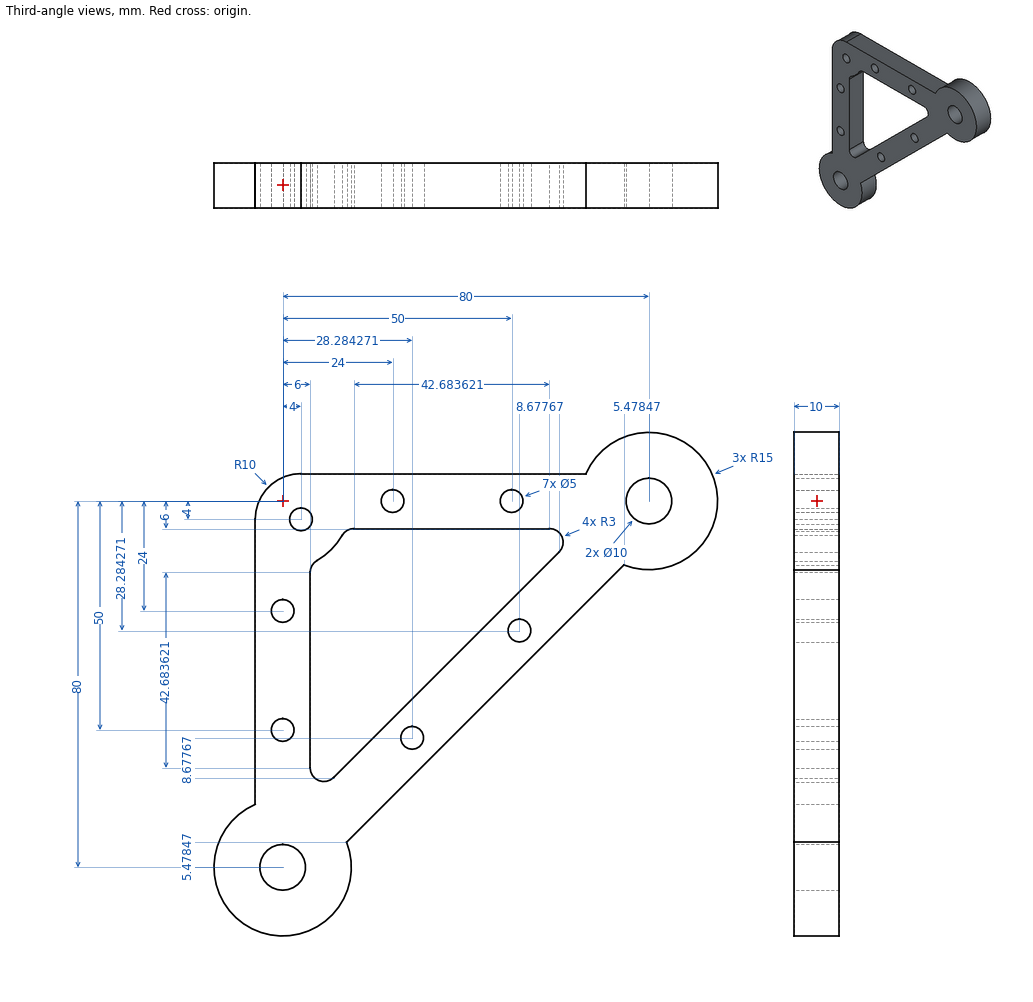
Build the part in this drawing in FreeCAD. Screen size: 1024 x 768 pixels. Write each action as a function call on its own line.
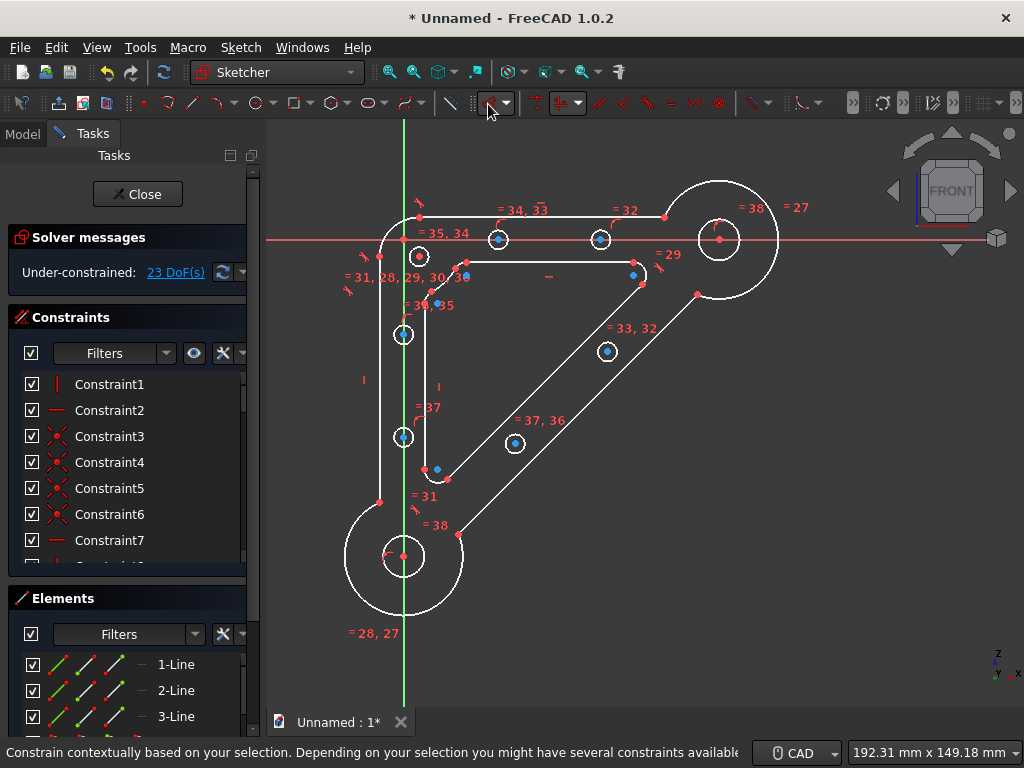
click(401, 222)
click(386, 194)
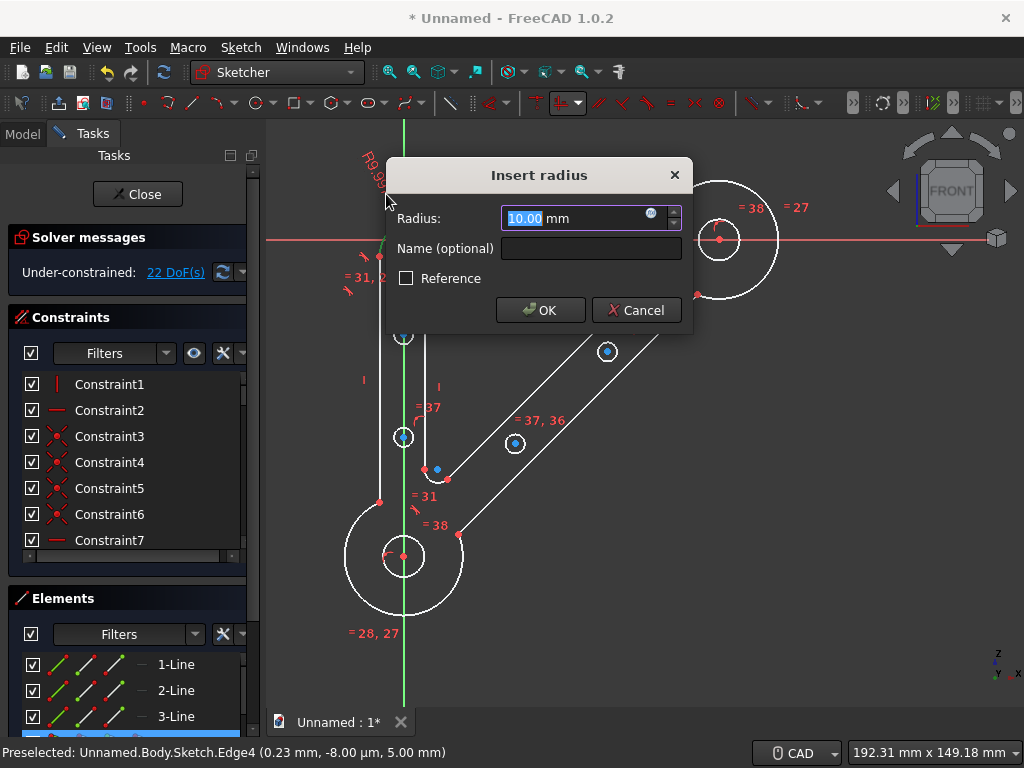
text(10)
key(Return)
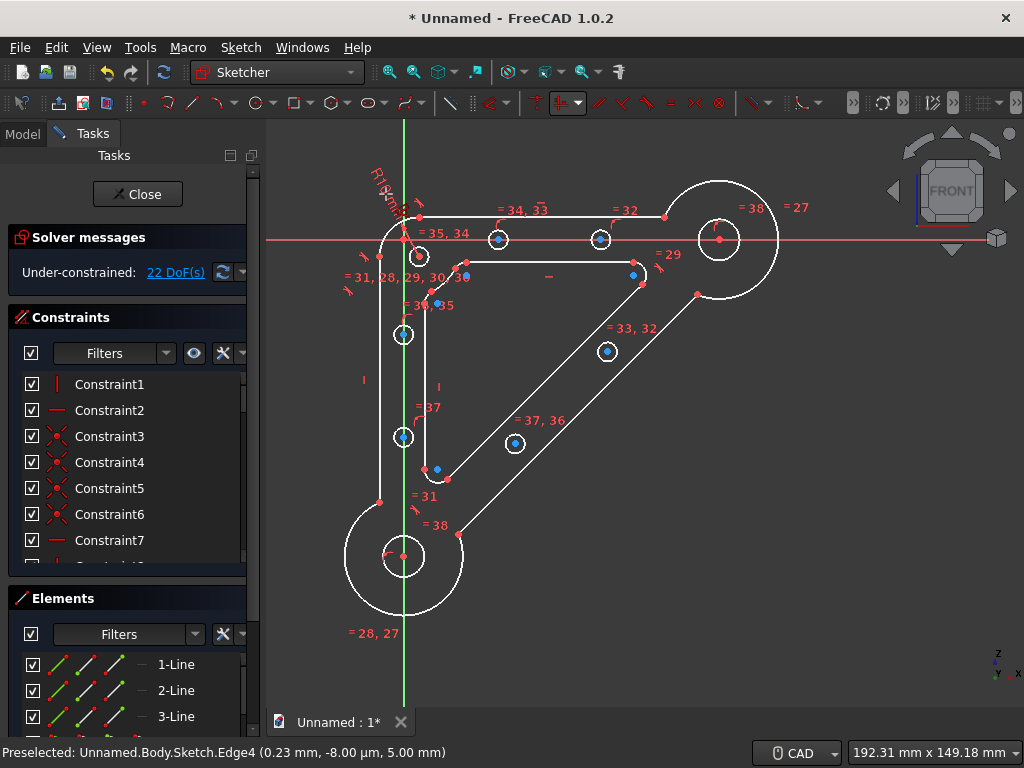
click(770, 270)
click(798, 286)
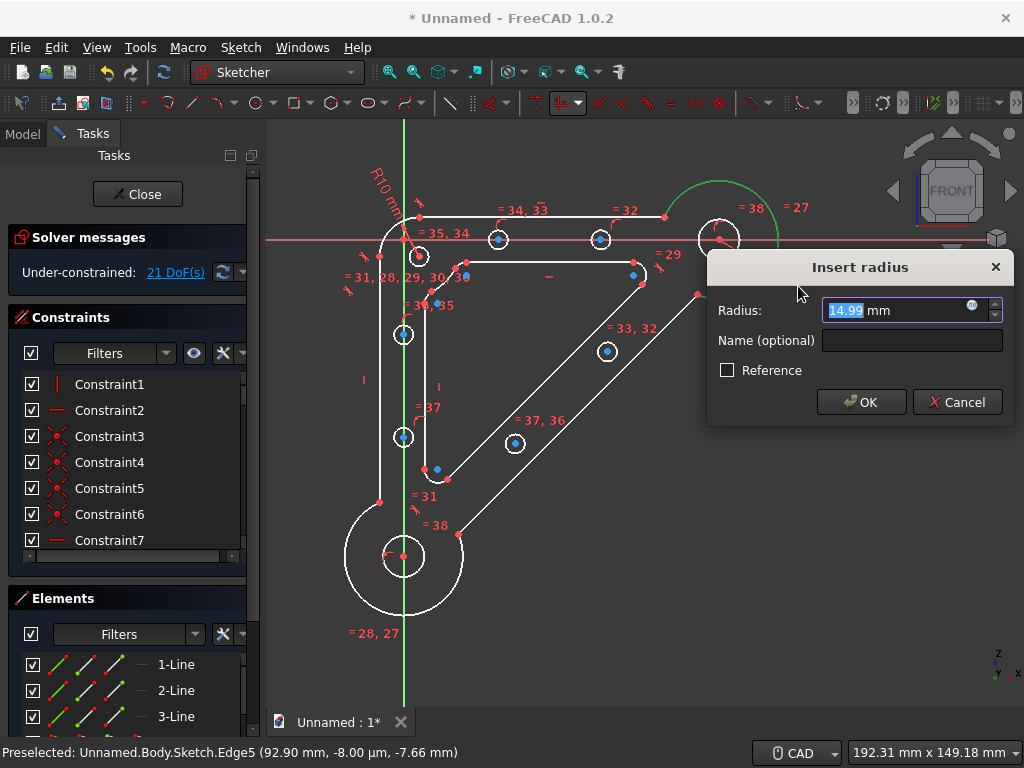
text(15)
key(Return)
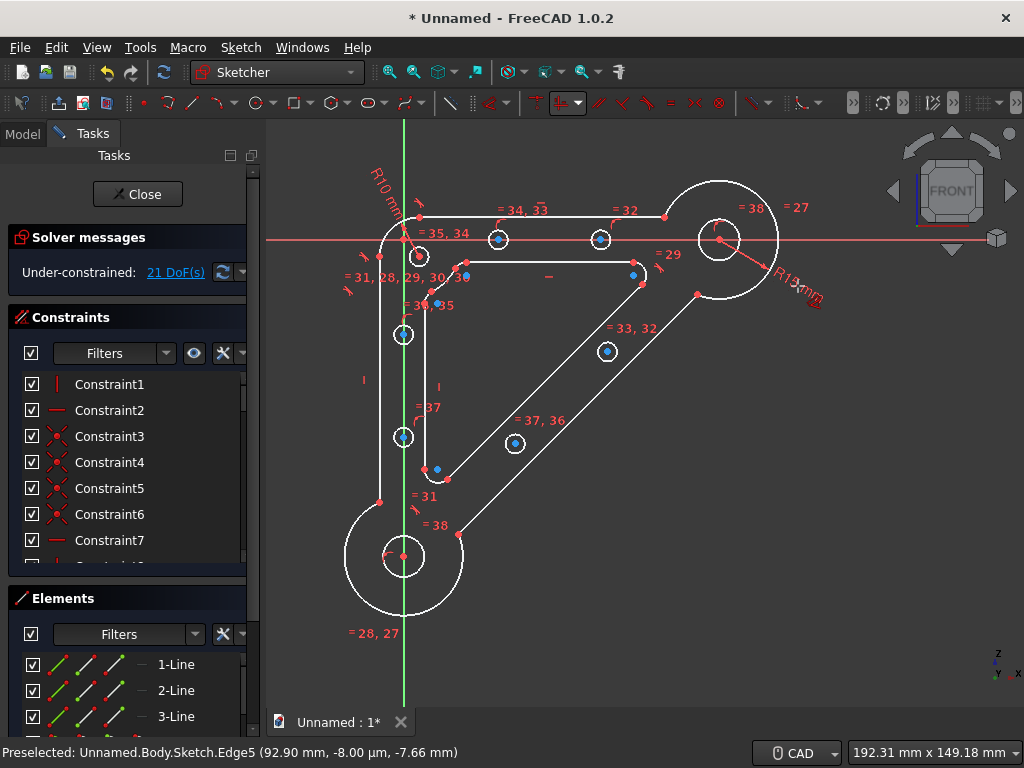
scroll(646, 276, up, 7)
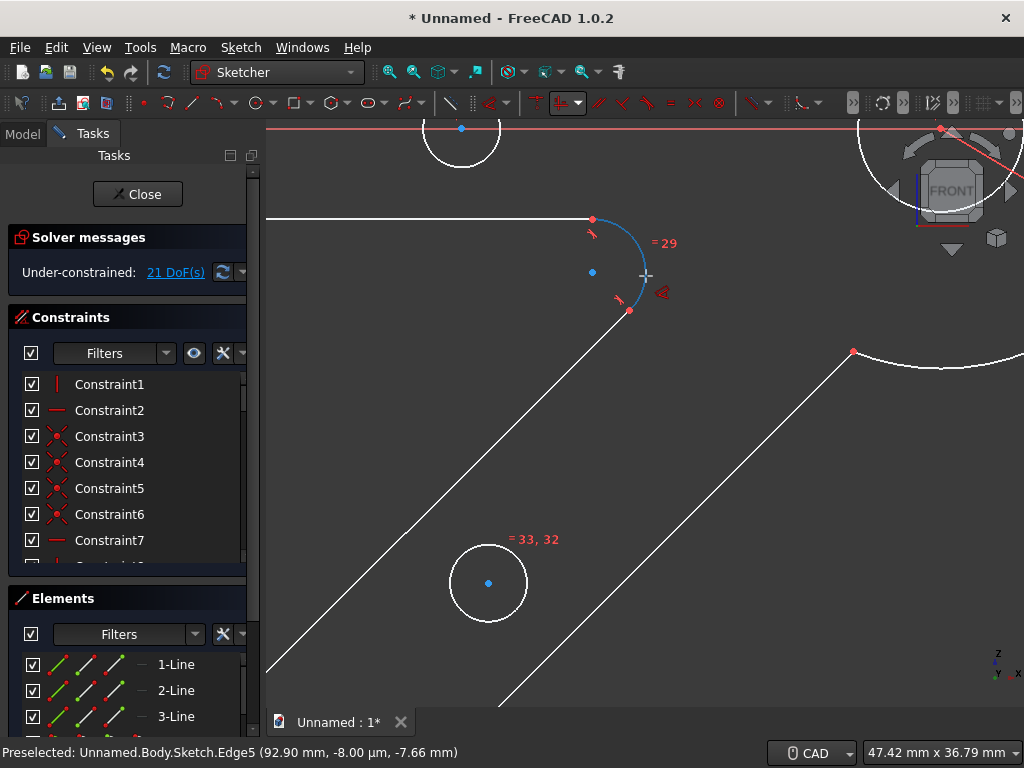
click(645, 277)
click(677, 280)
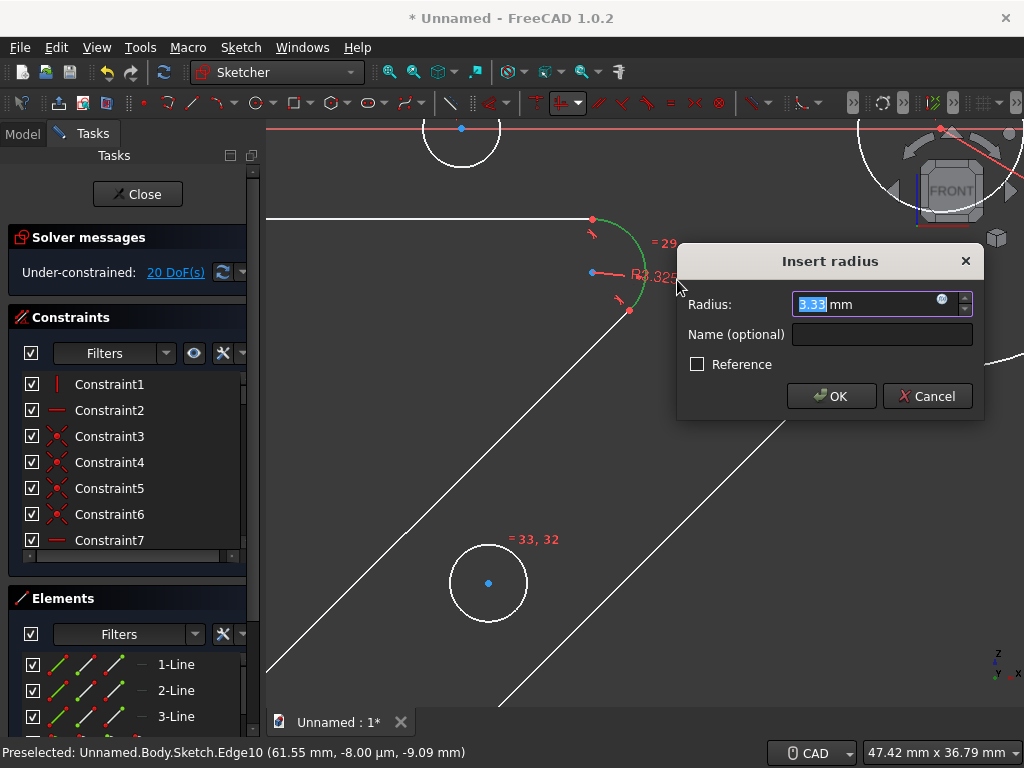
text(3)
key(Return)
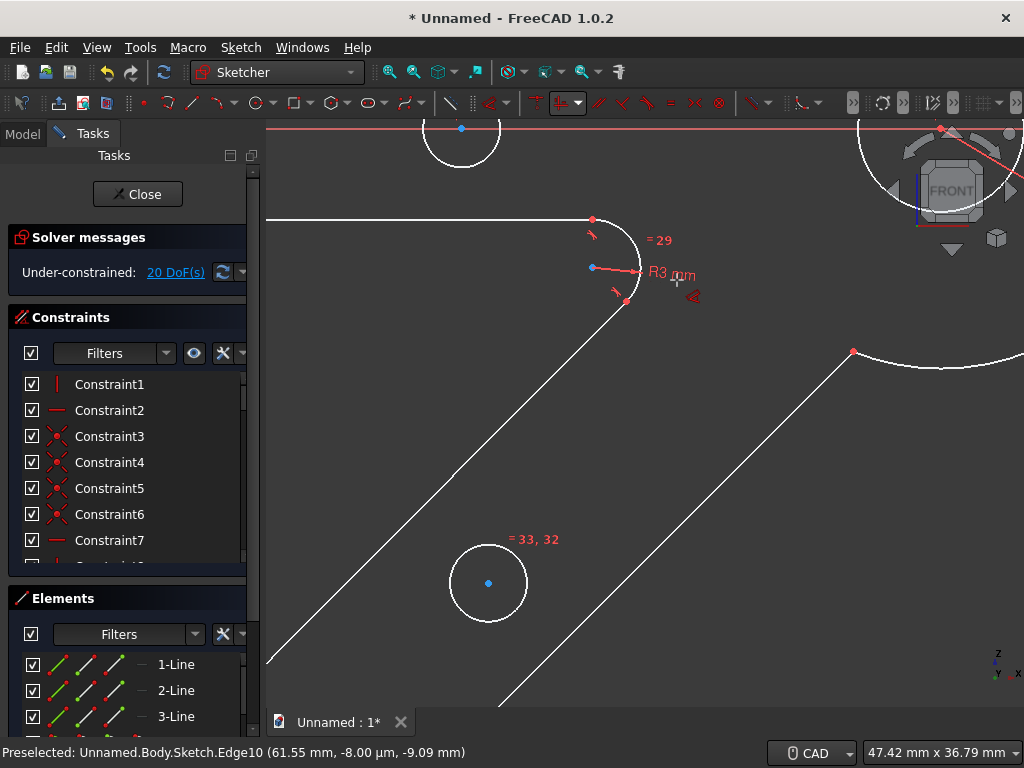
scroll(646, 276, down, 7)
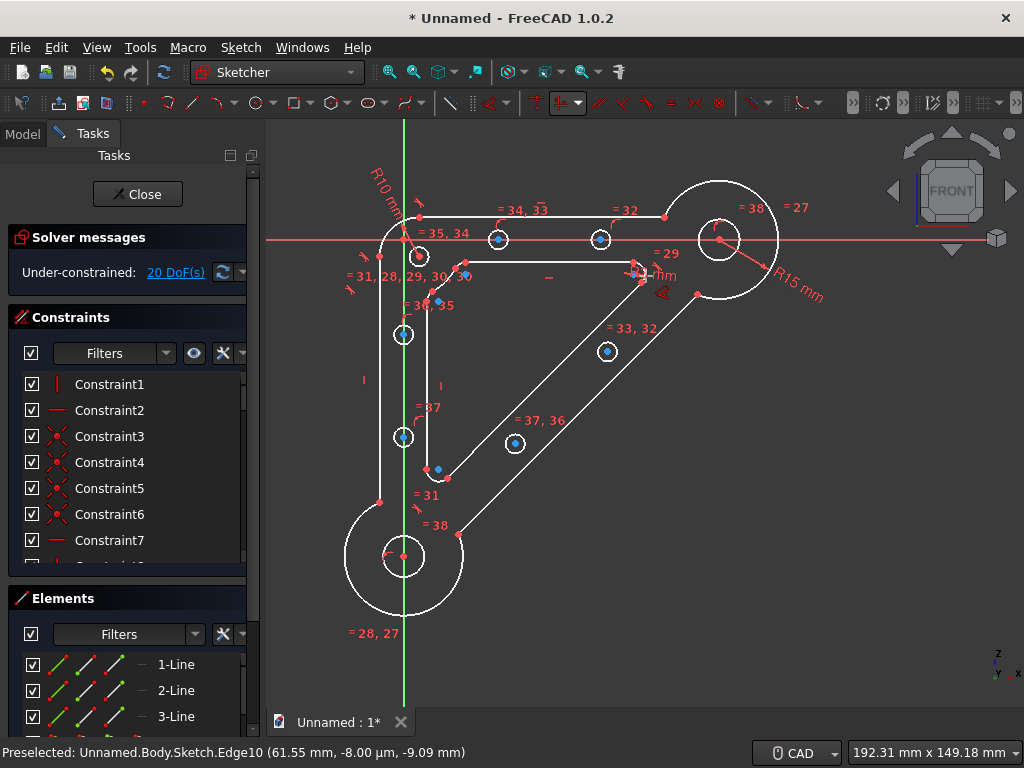
click(734, 225)
click(773, 186)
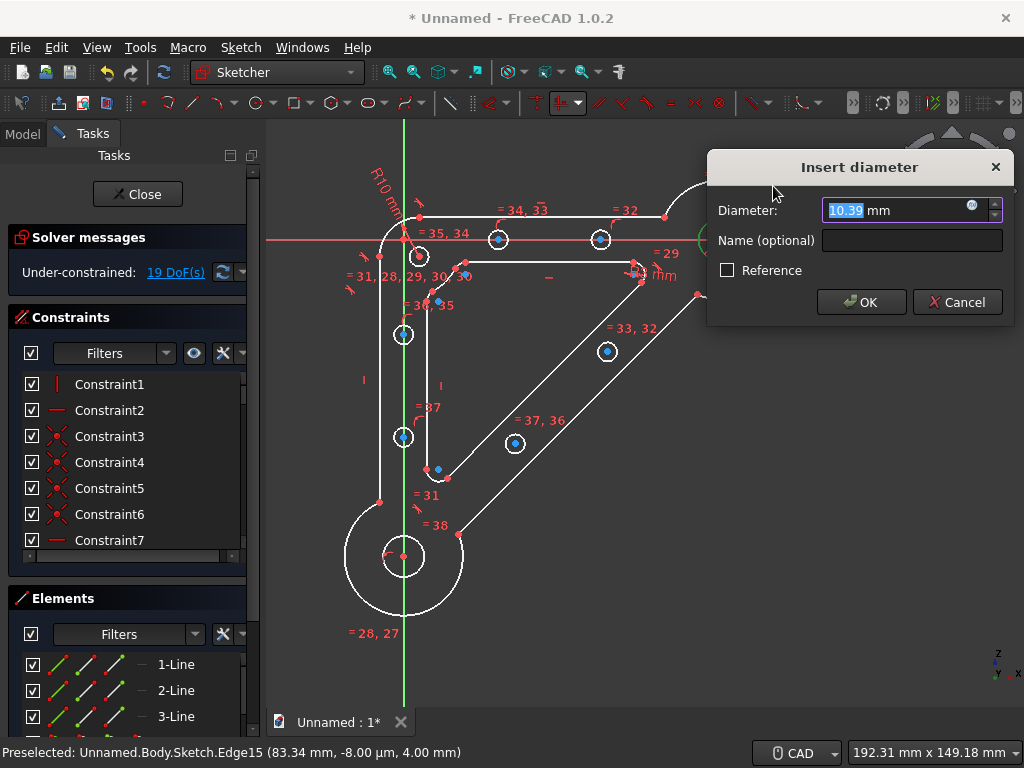
text(10)
key(Return)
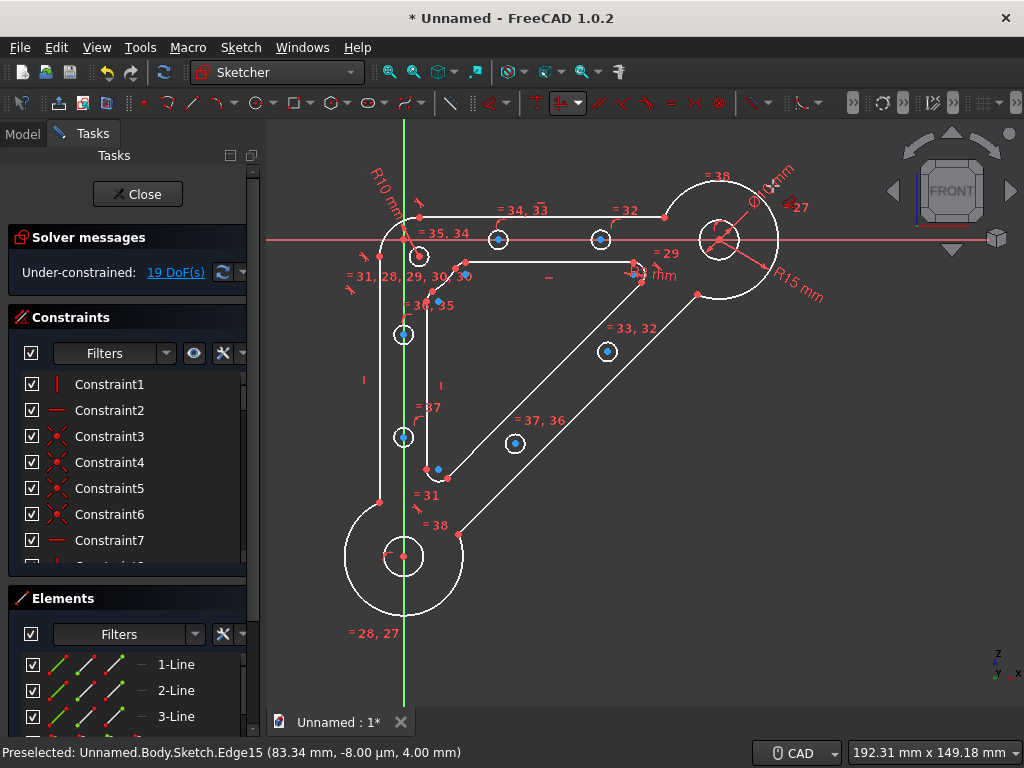
scroll(601, 230, up, 4)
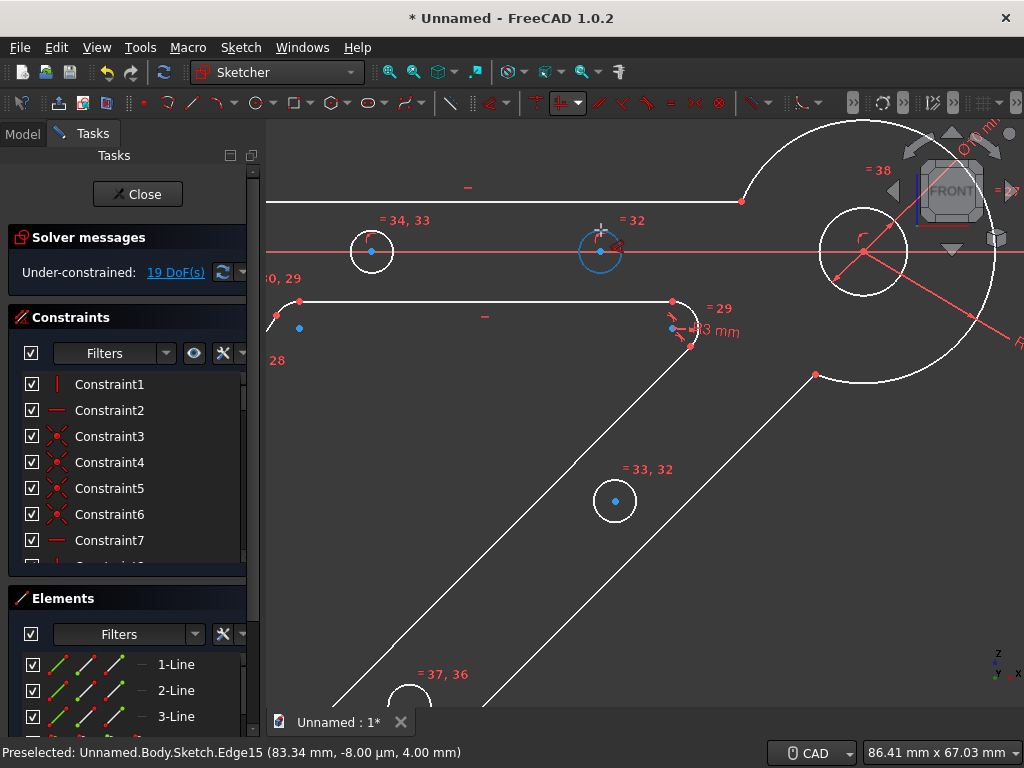
click(601, 231)
click(646, 225)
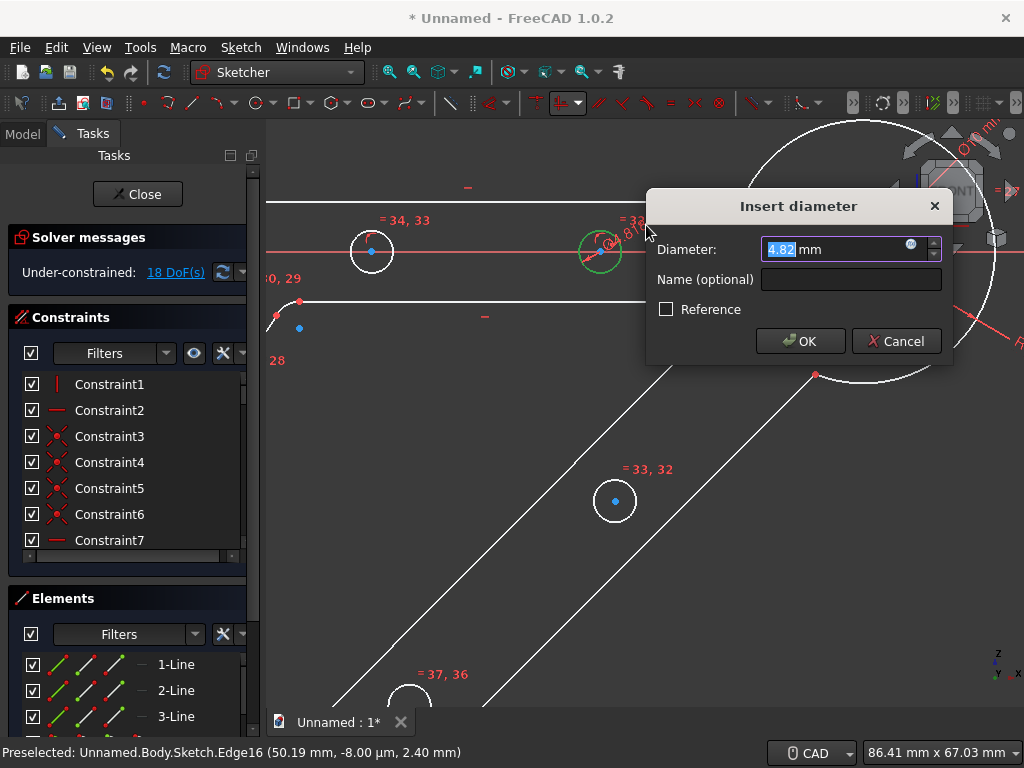
text(5)
key(Return)